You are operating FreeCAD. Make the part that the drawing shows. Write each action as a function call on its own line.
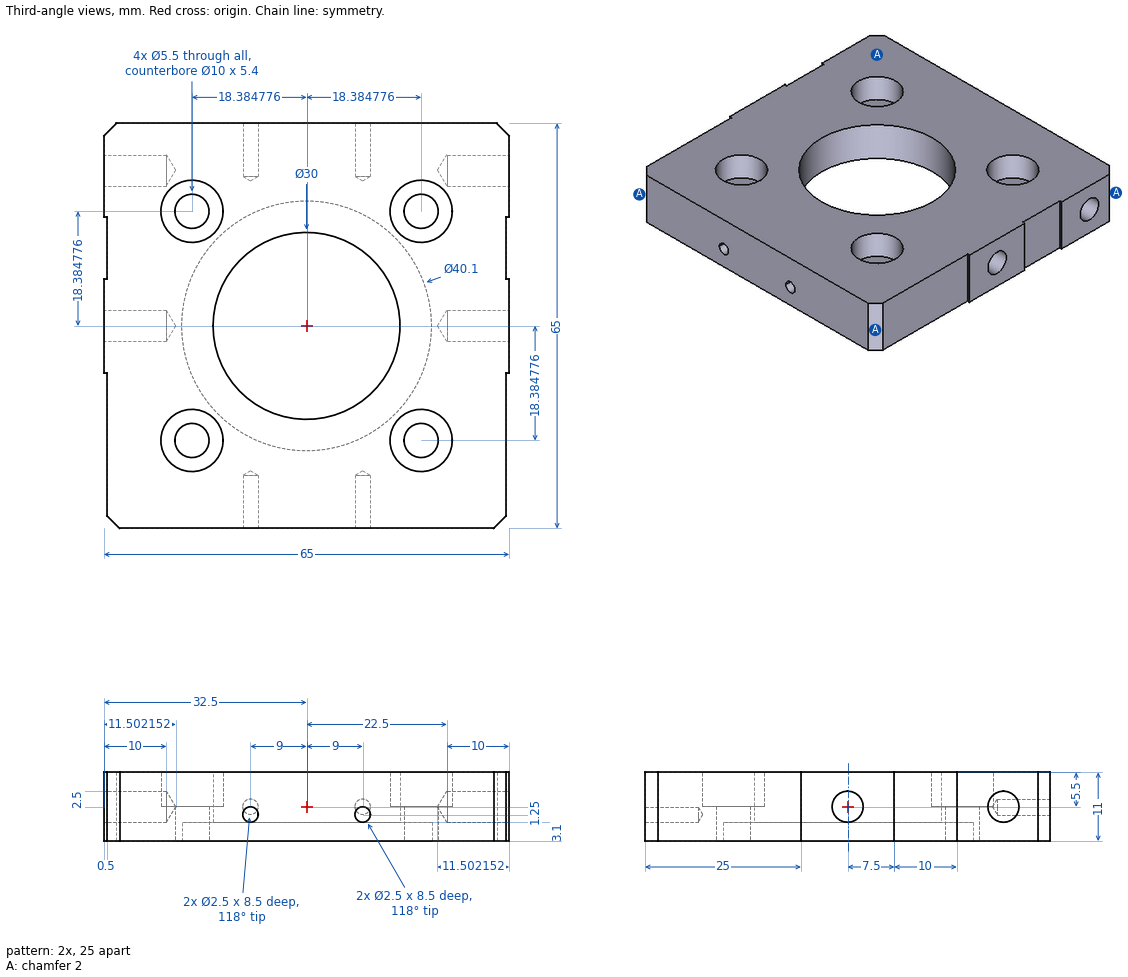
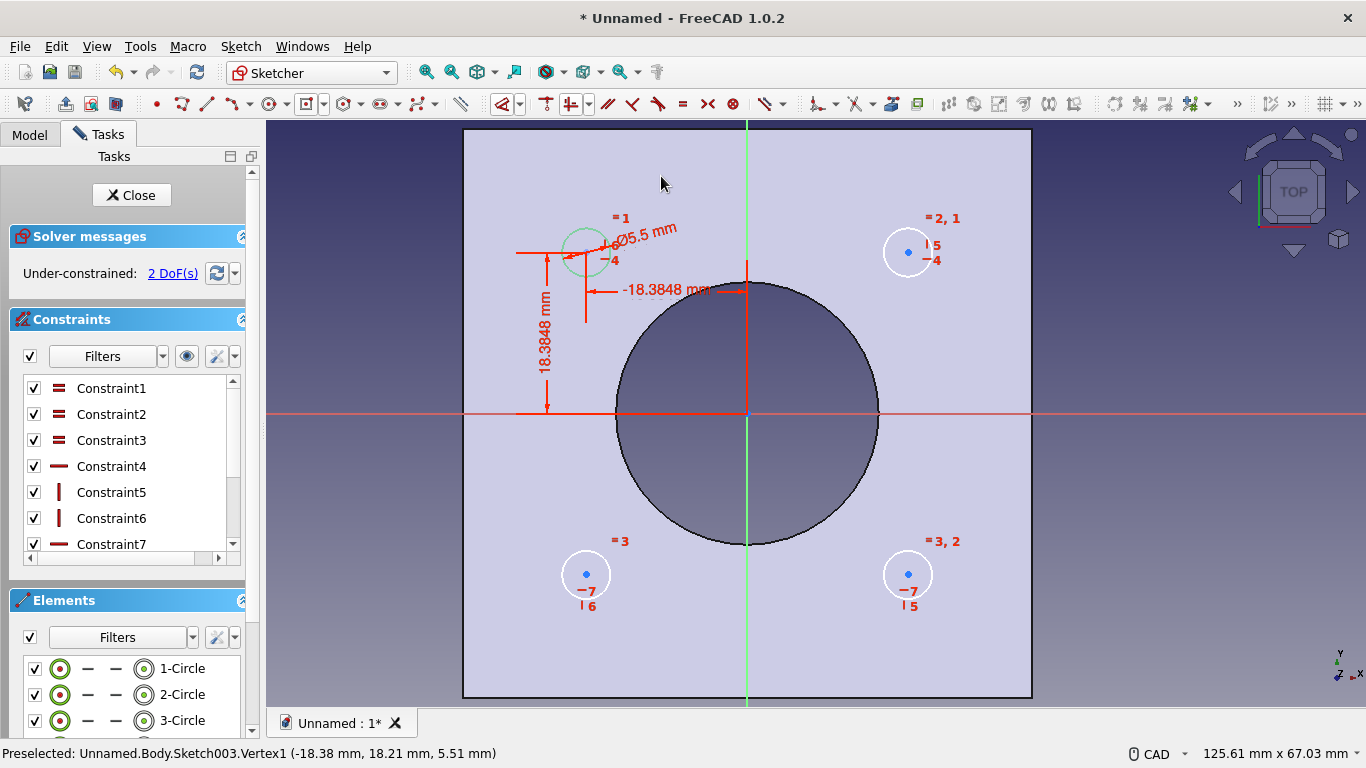
click(908, 253)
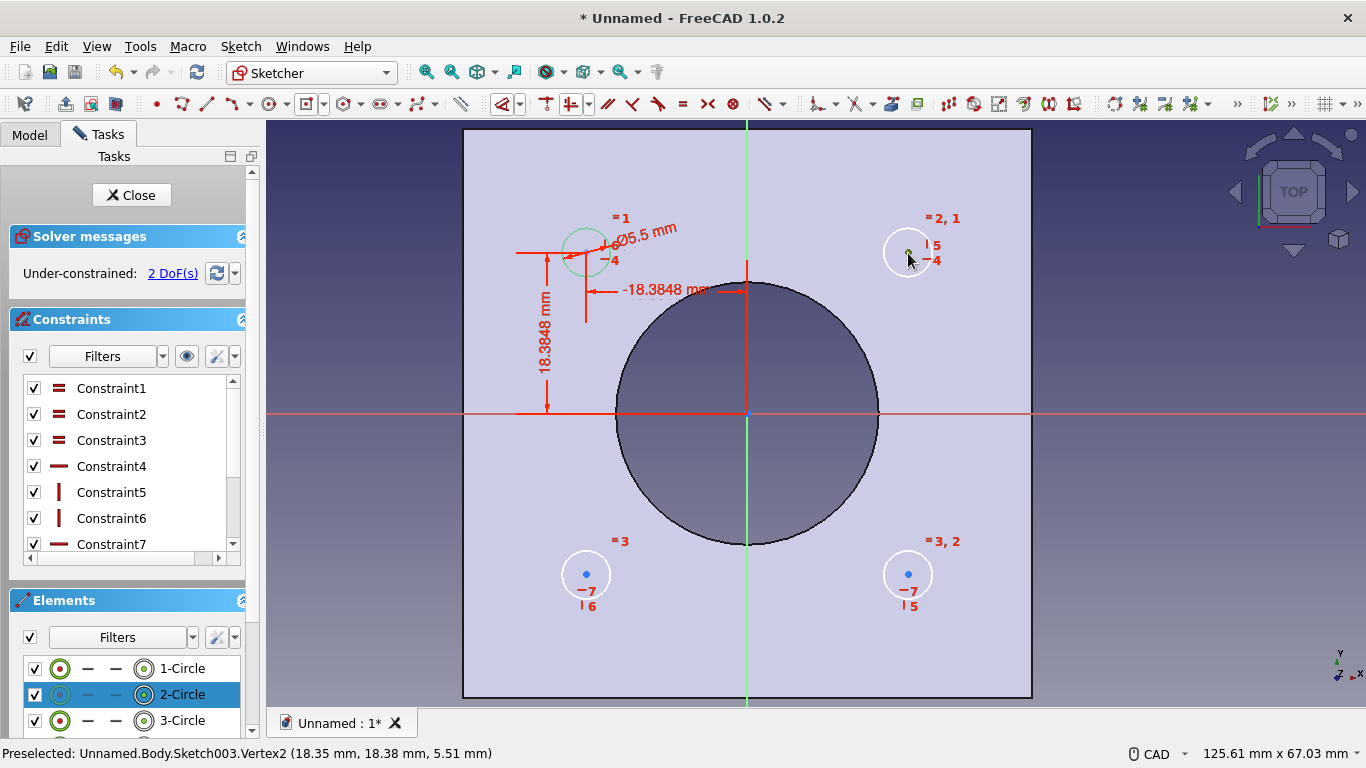
key(l)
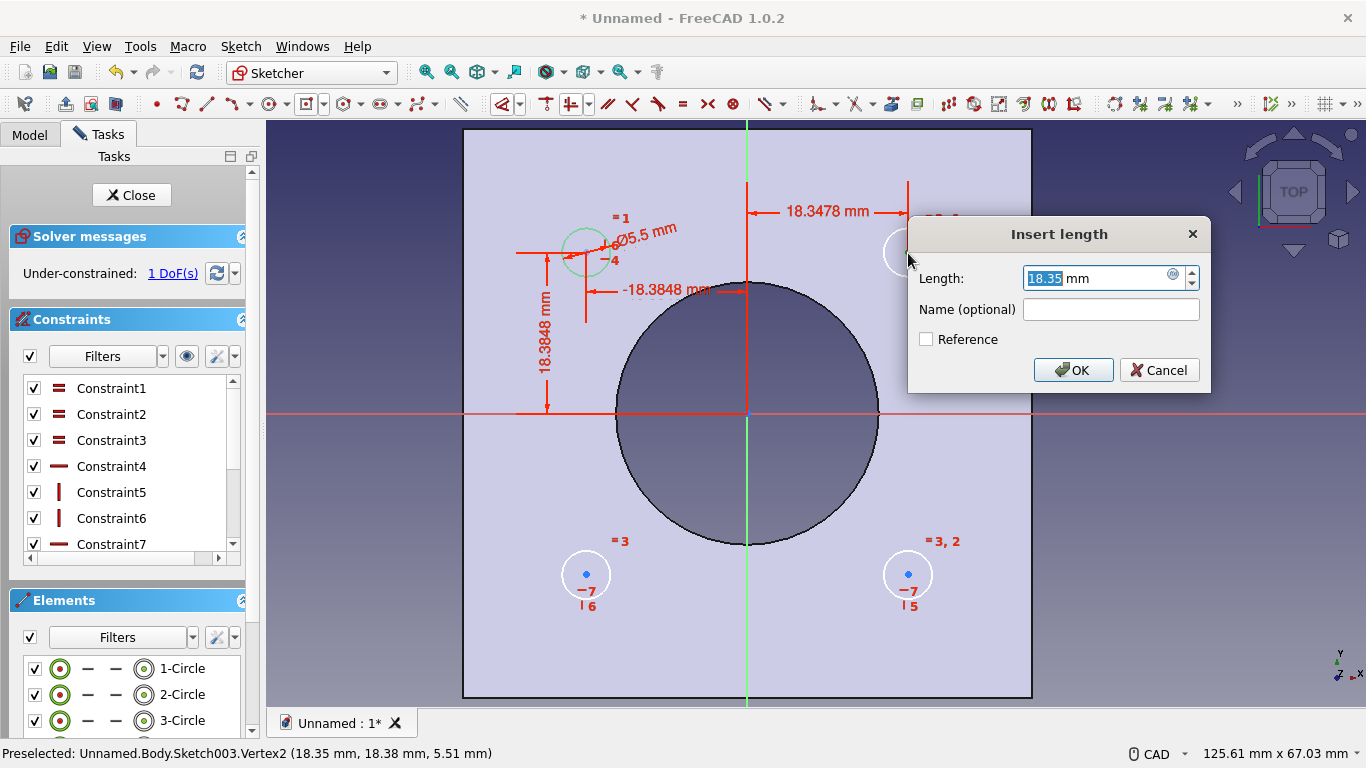
text(18.384776)
key(Return)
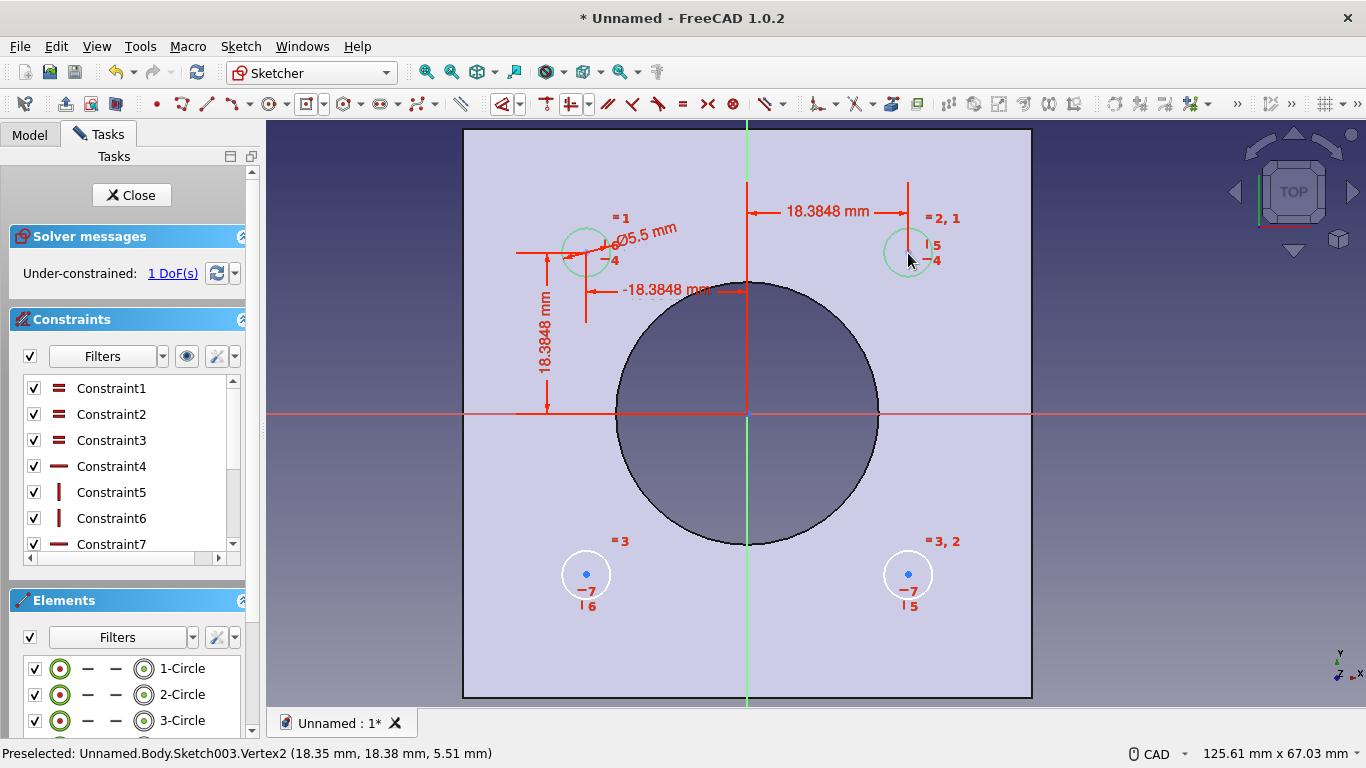
click(908, 575)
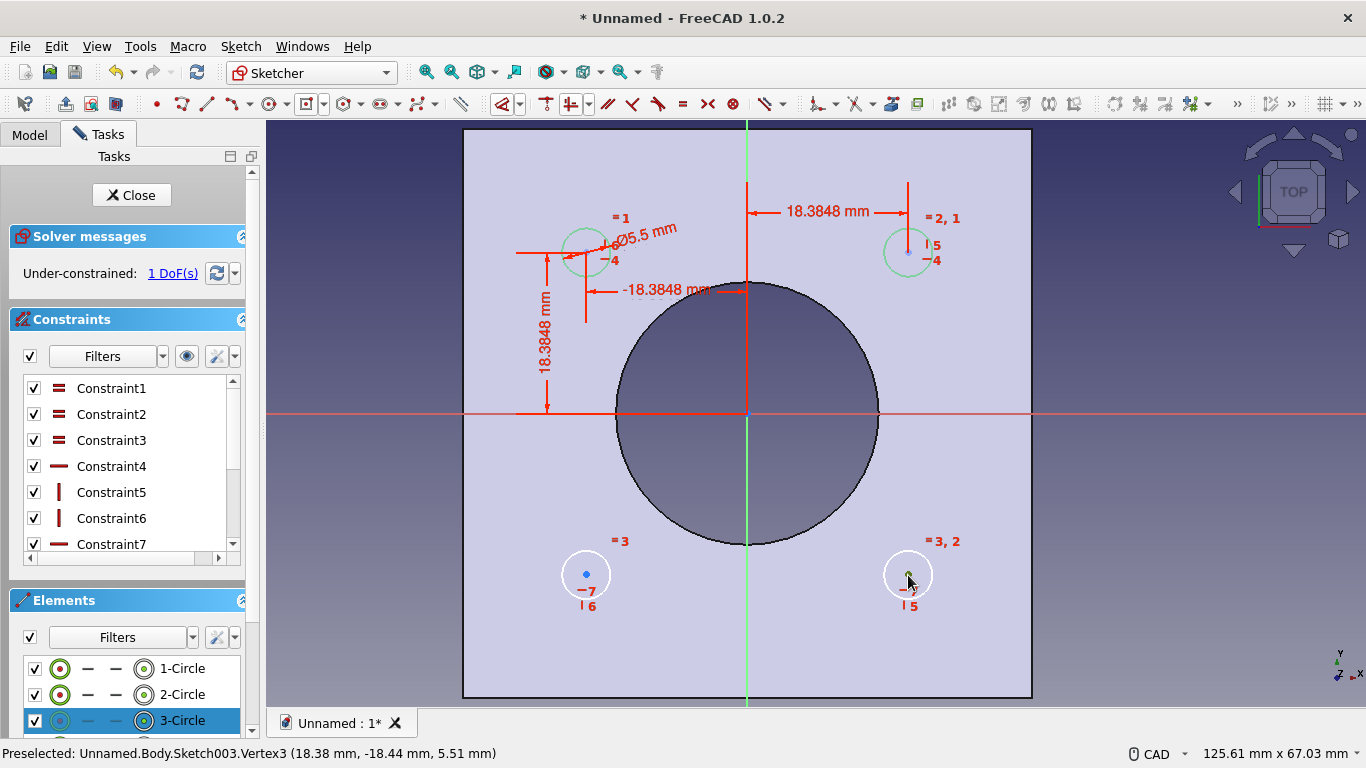
click(520, 104)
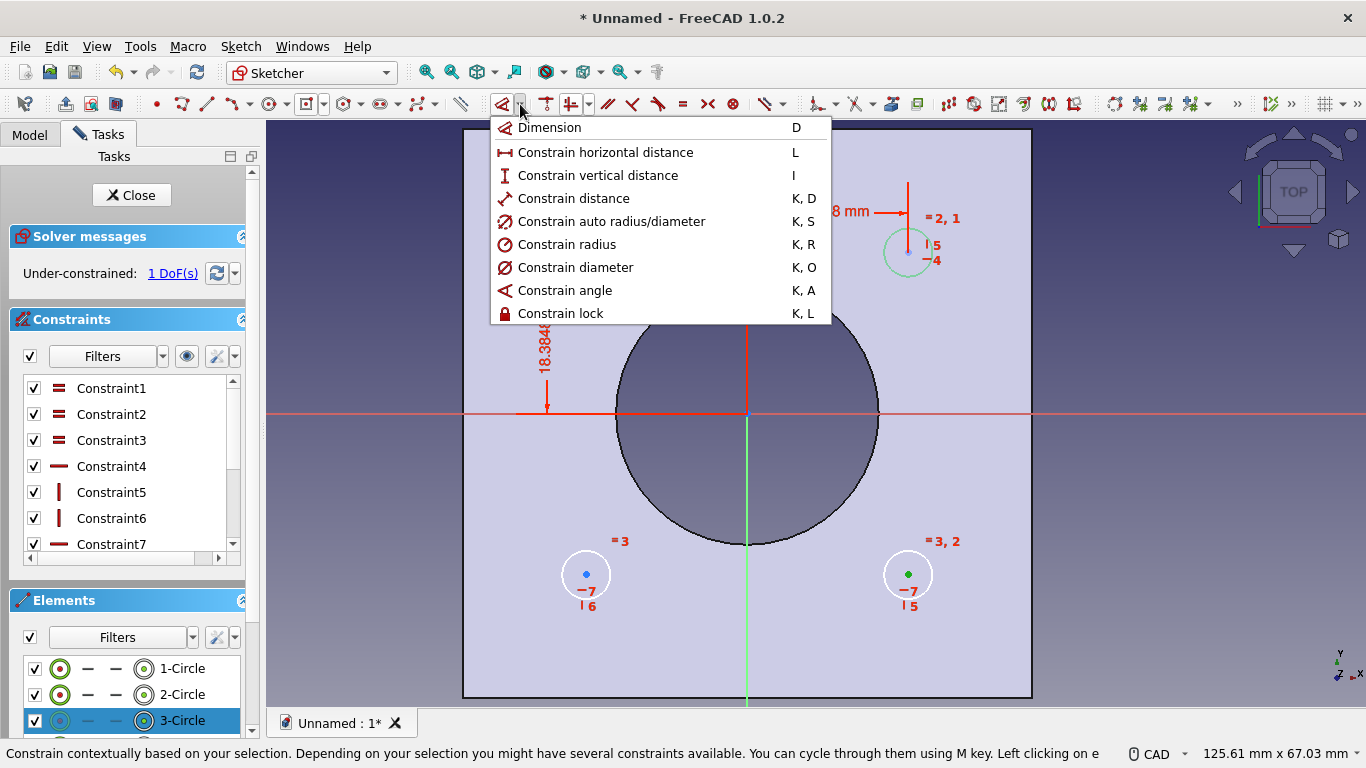
click(661, 176)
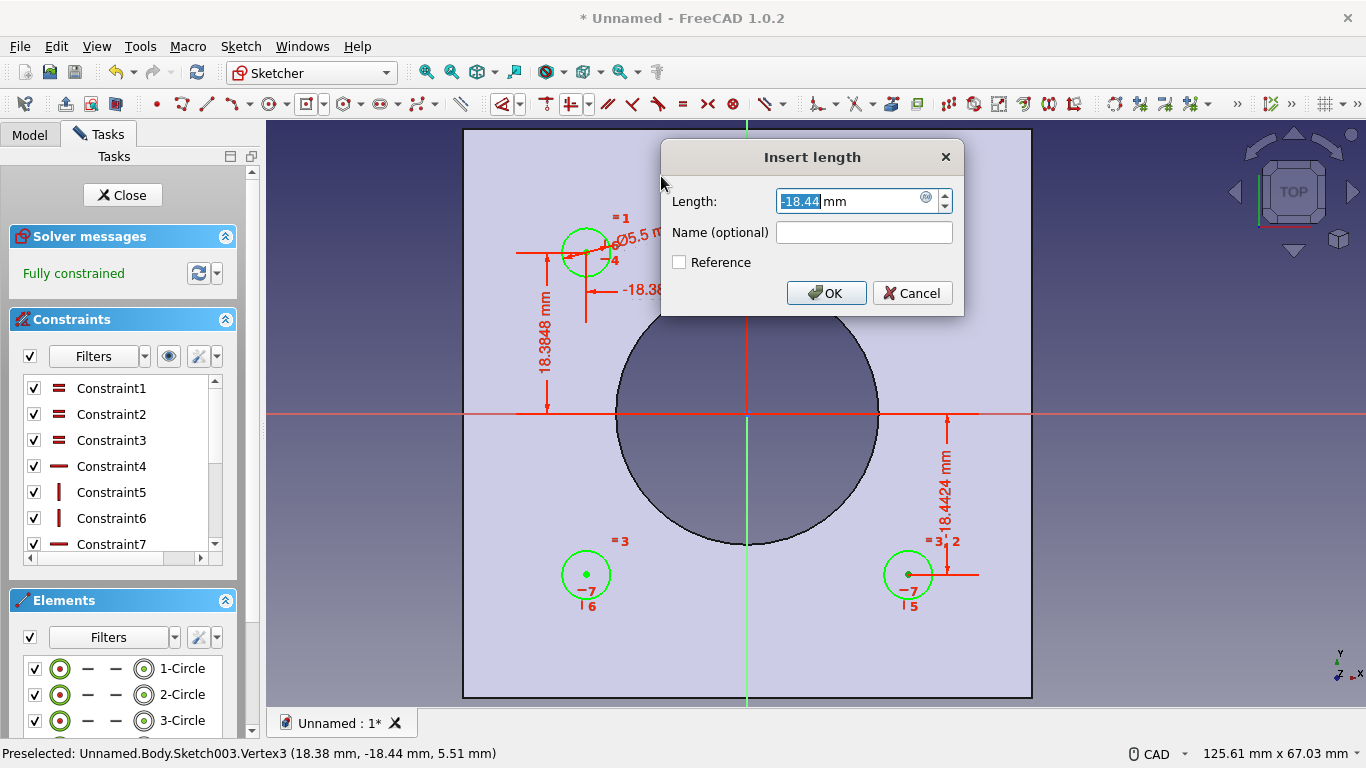
text(-18.384776)
key(Return)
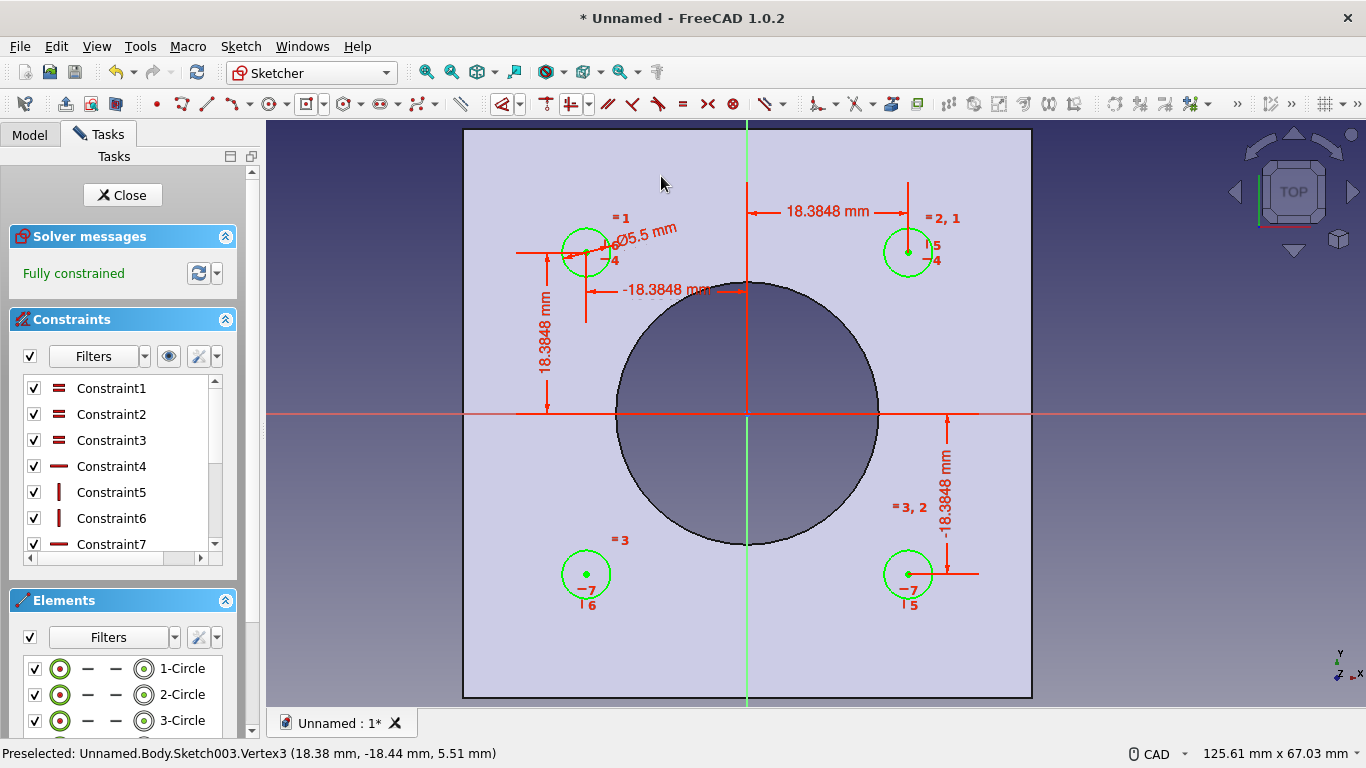
click(123, 195)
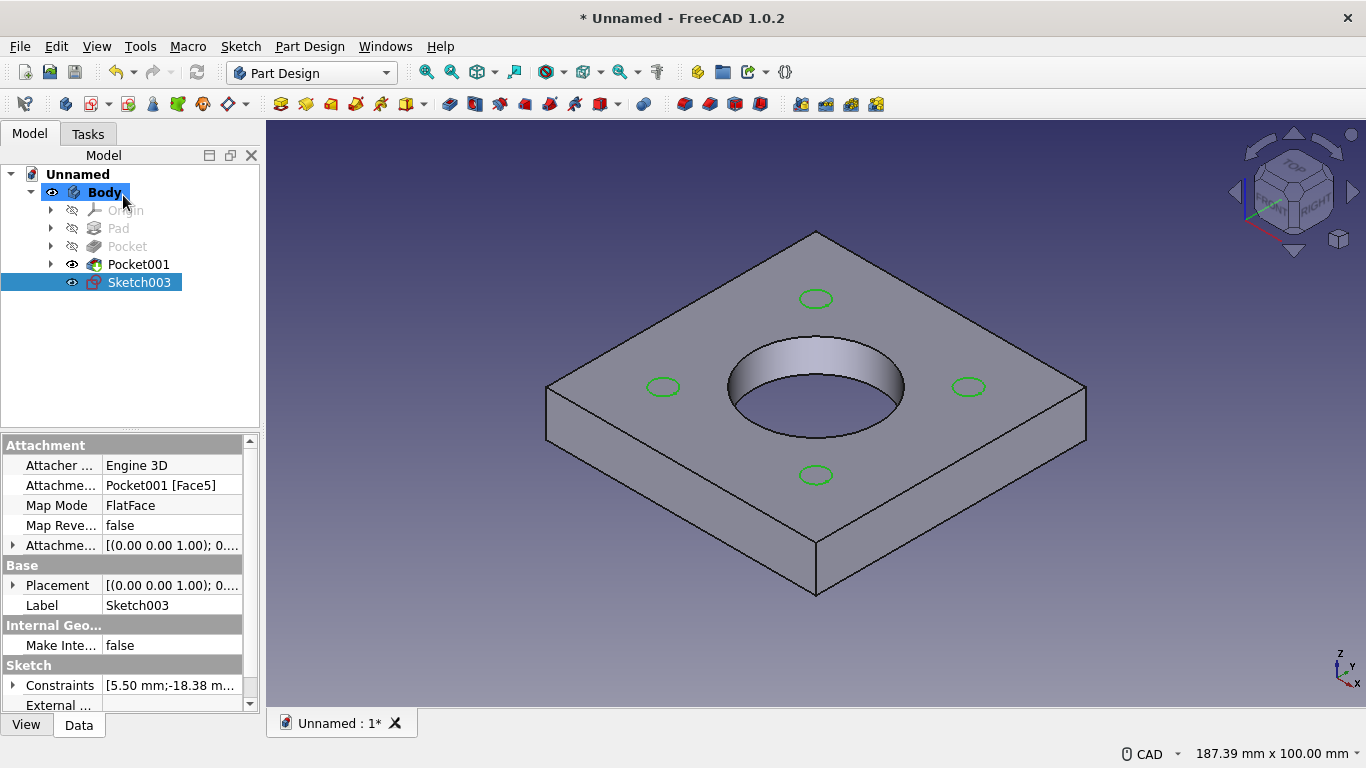
click(475, 104)